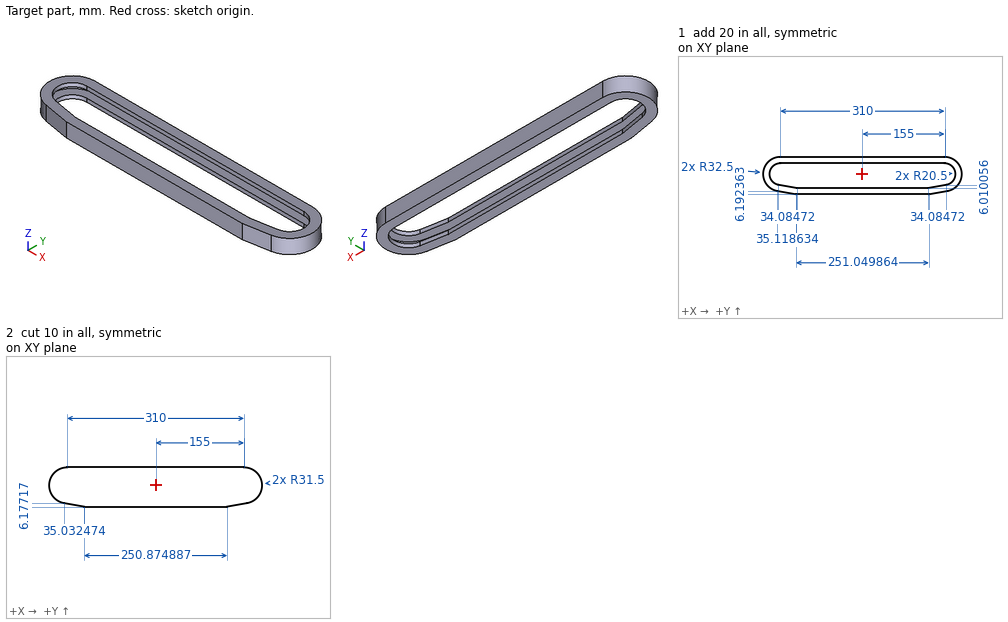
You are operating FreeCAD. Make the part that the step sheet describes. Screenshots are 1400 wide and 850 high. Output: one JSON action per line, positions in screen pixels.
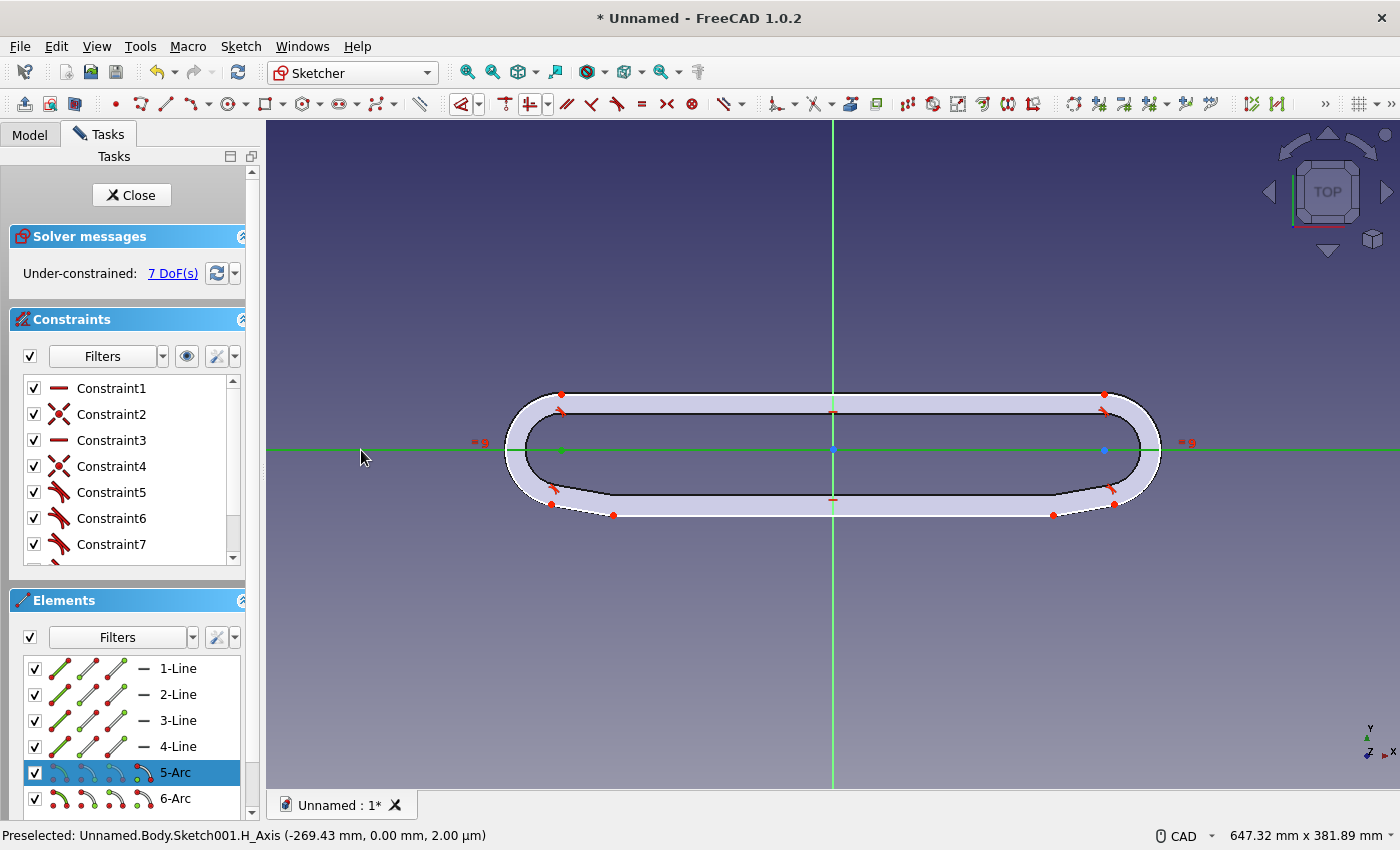
{"action": "left_click", "coordinate": [505, 104]}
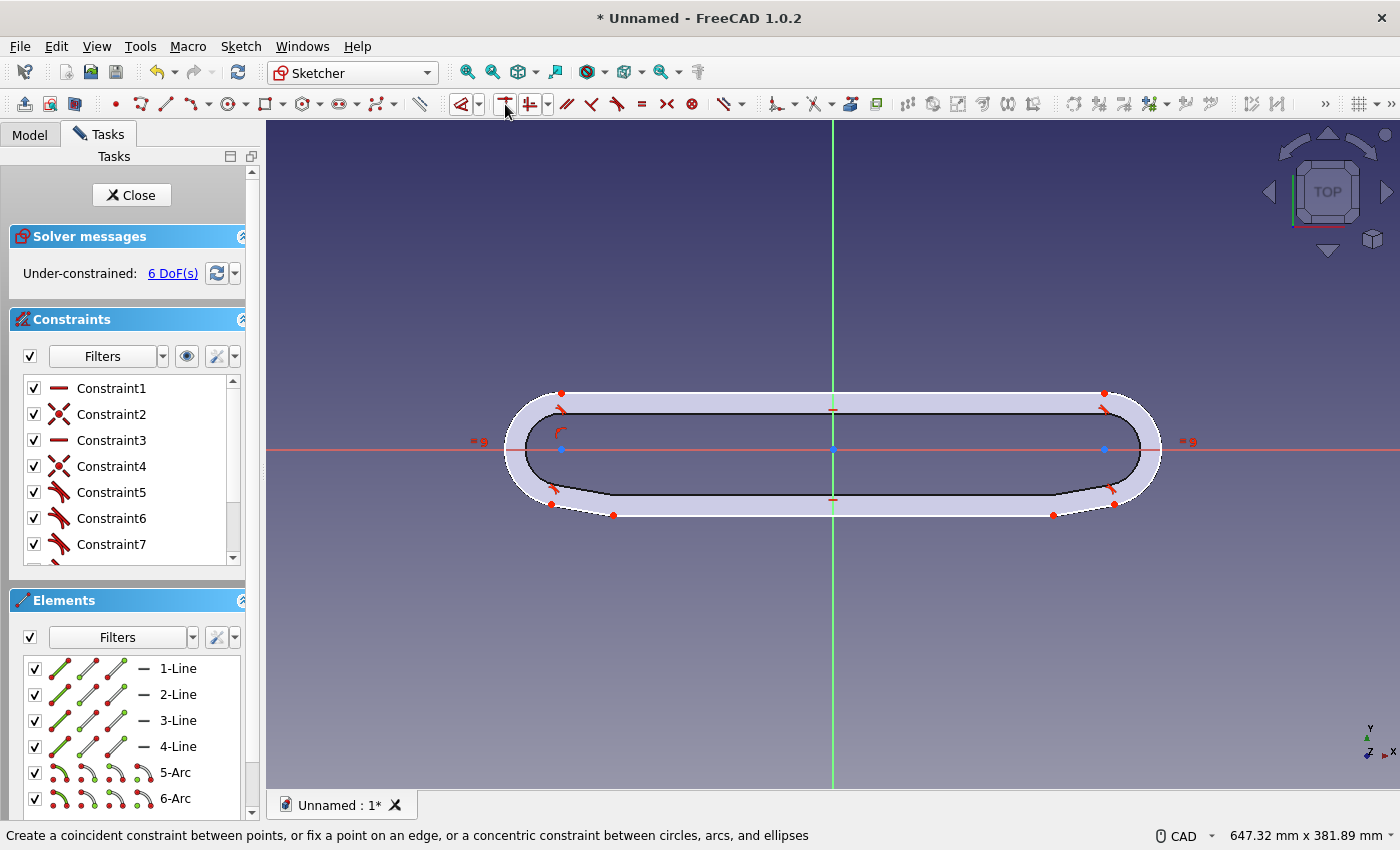
{"action": "left_click", "coordinate": [518, 414]}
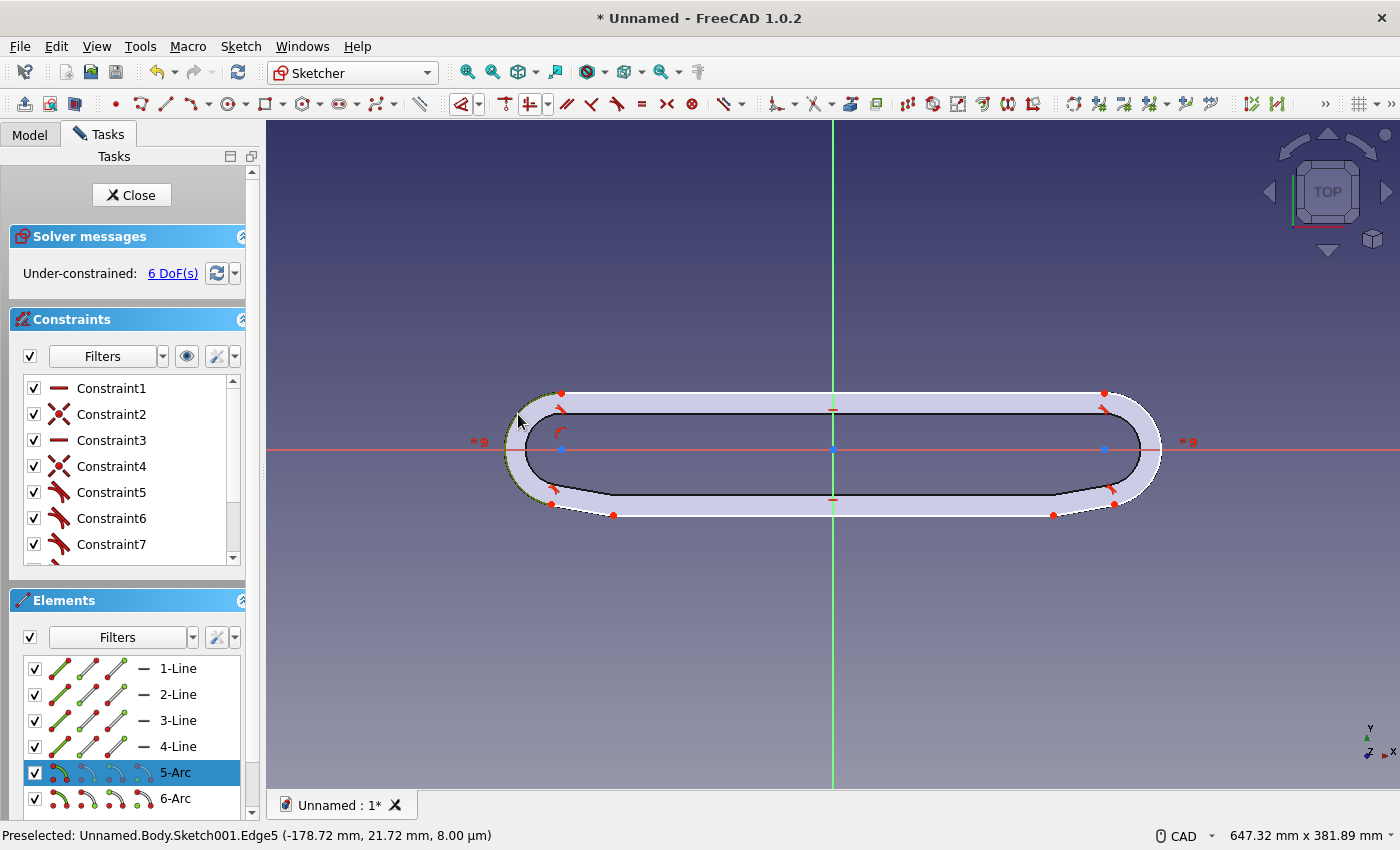
{"action": "key", "text": "k r"}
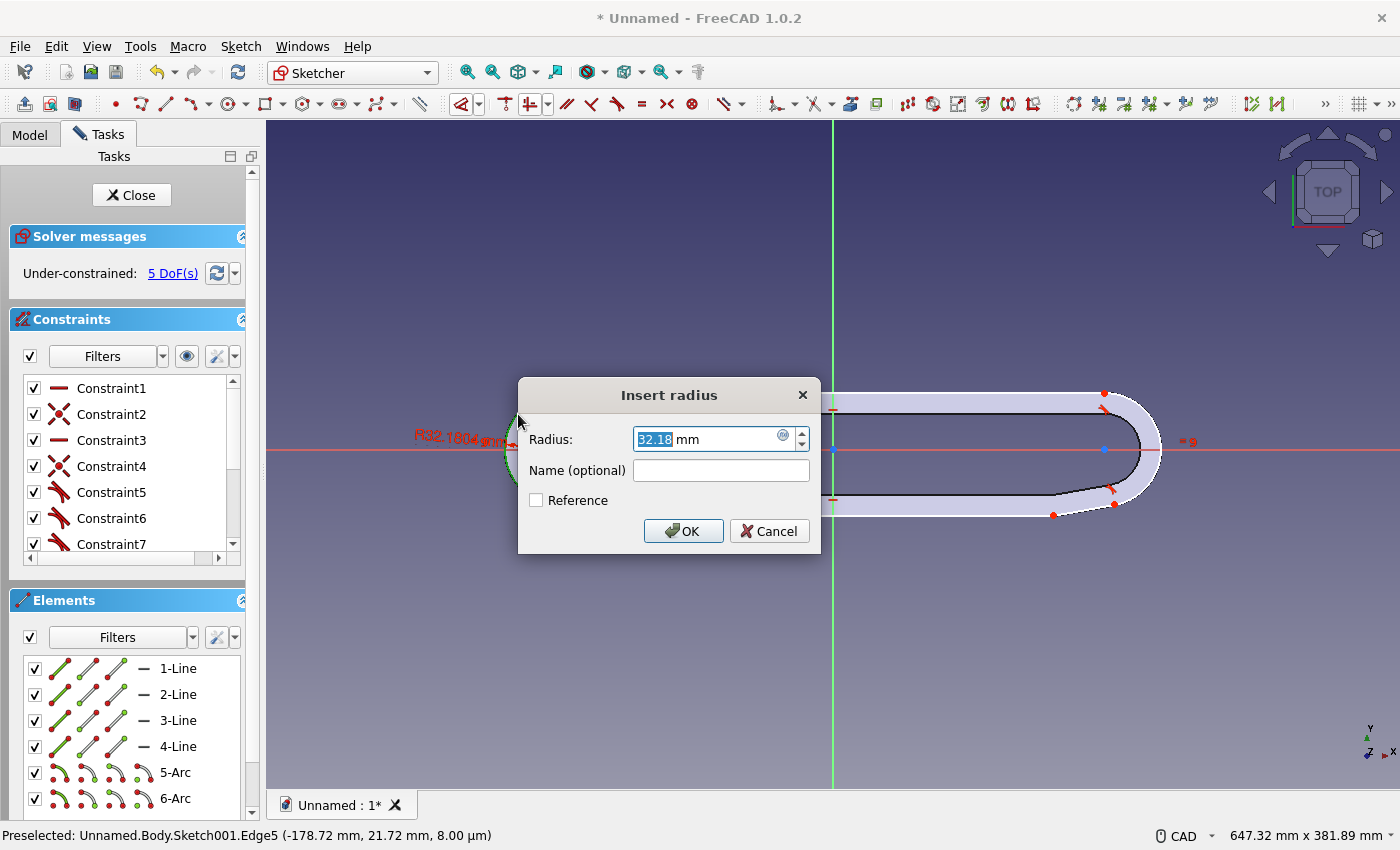
{"action": "type", "text": "31.5"}
{"action": "key", "text": "Return"}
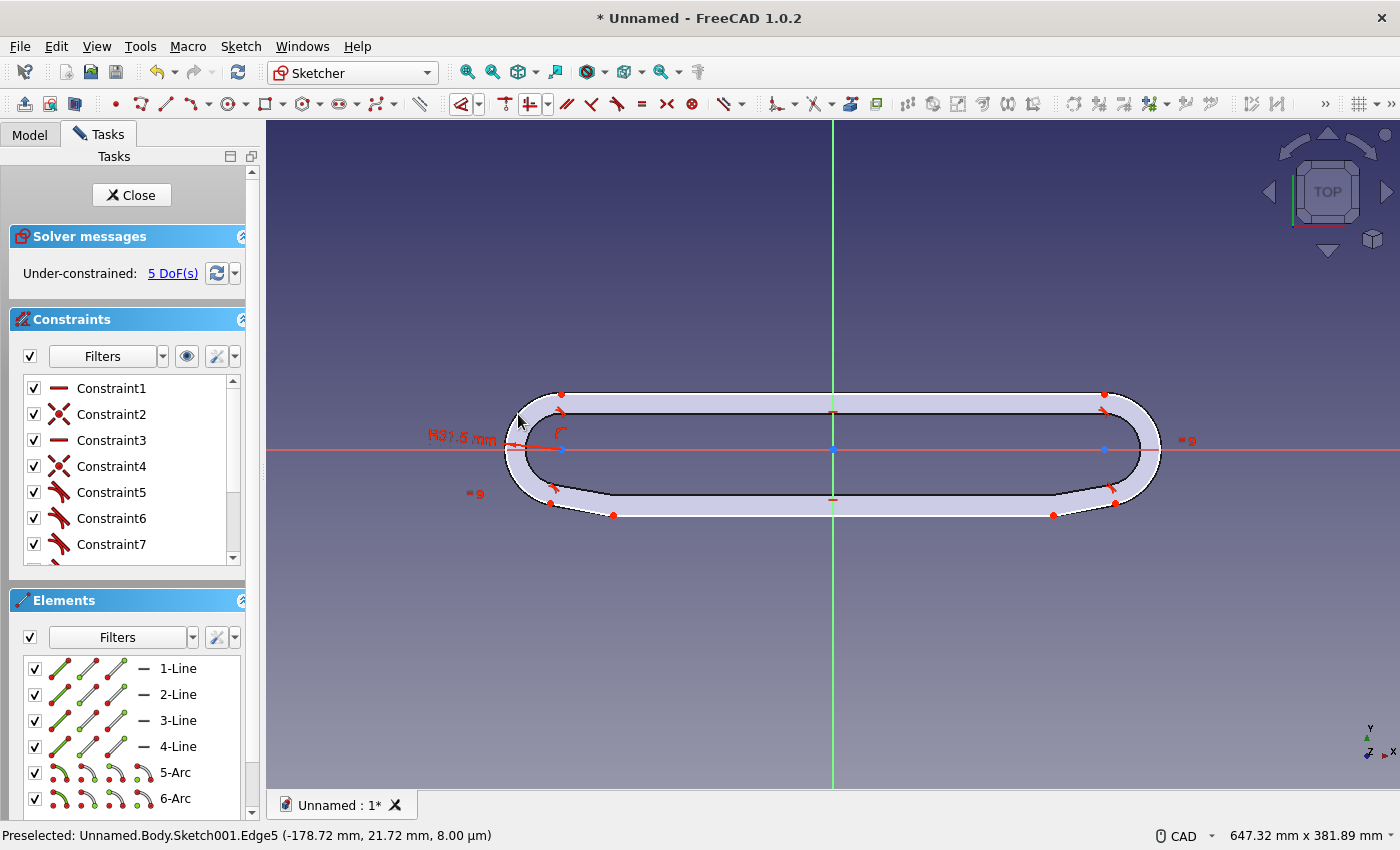
{"action": "left_click", "coordinate": [942, 394]}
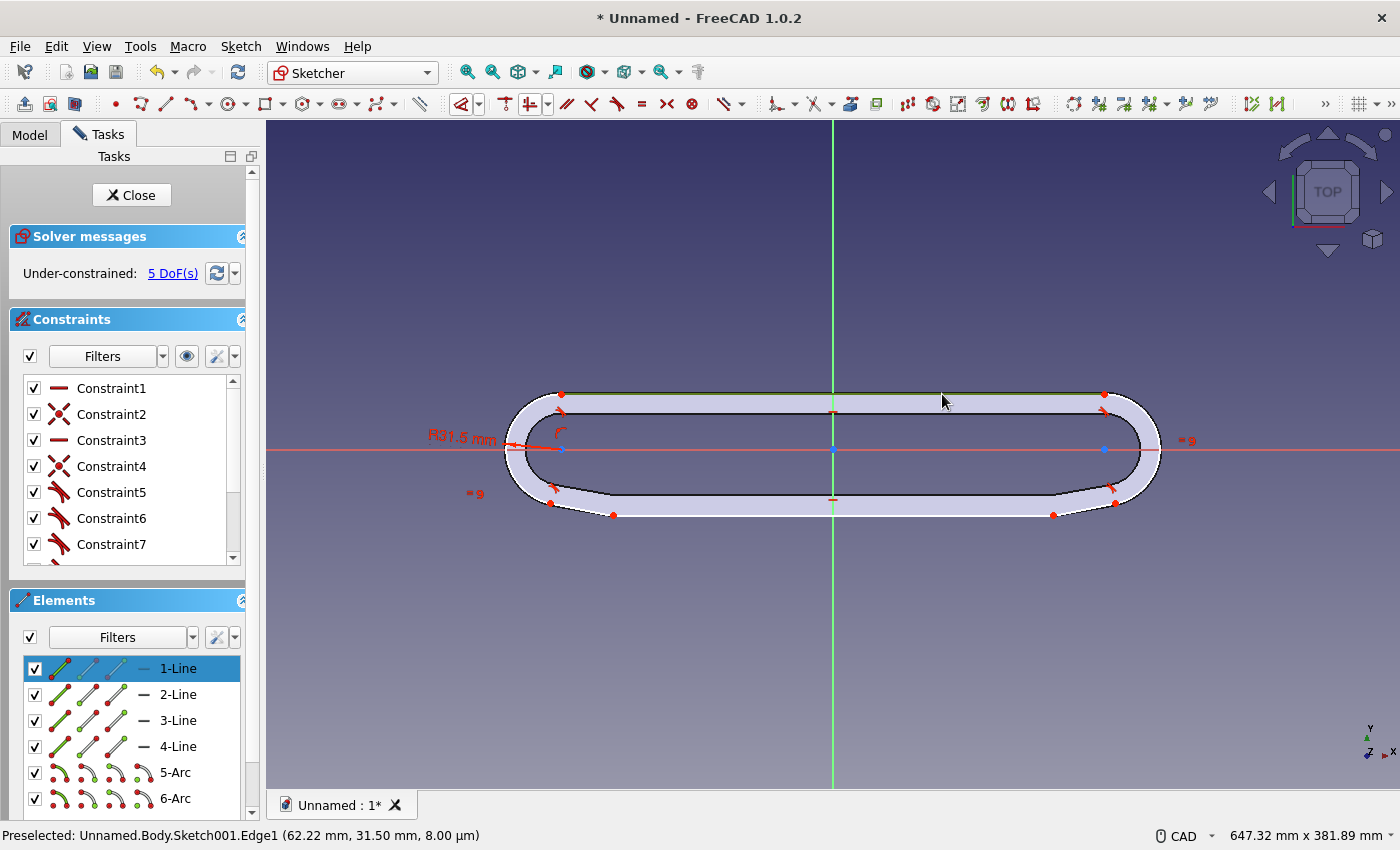
{"action": "key", "text": "l"}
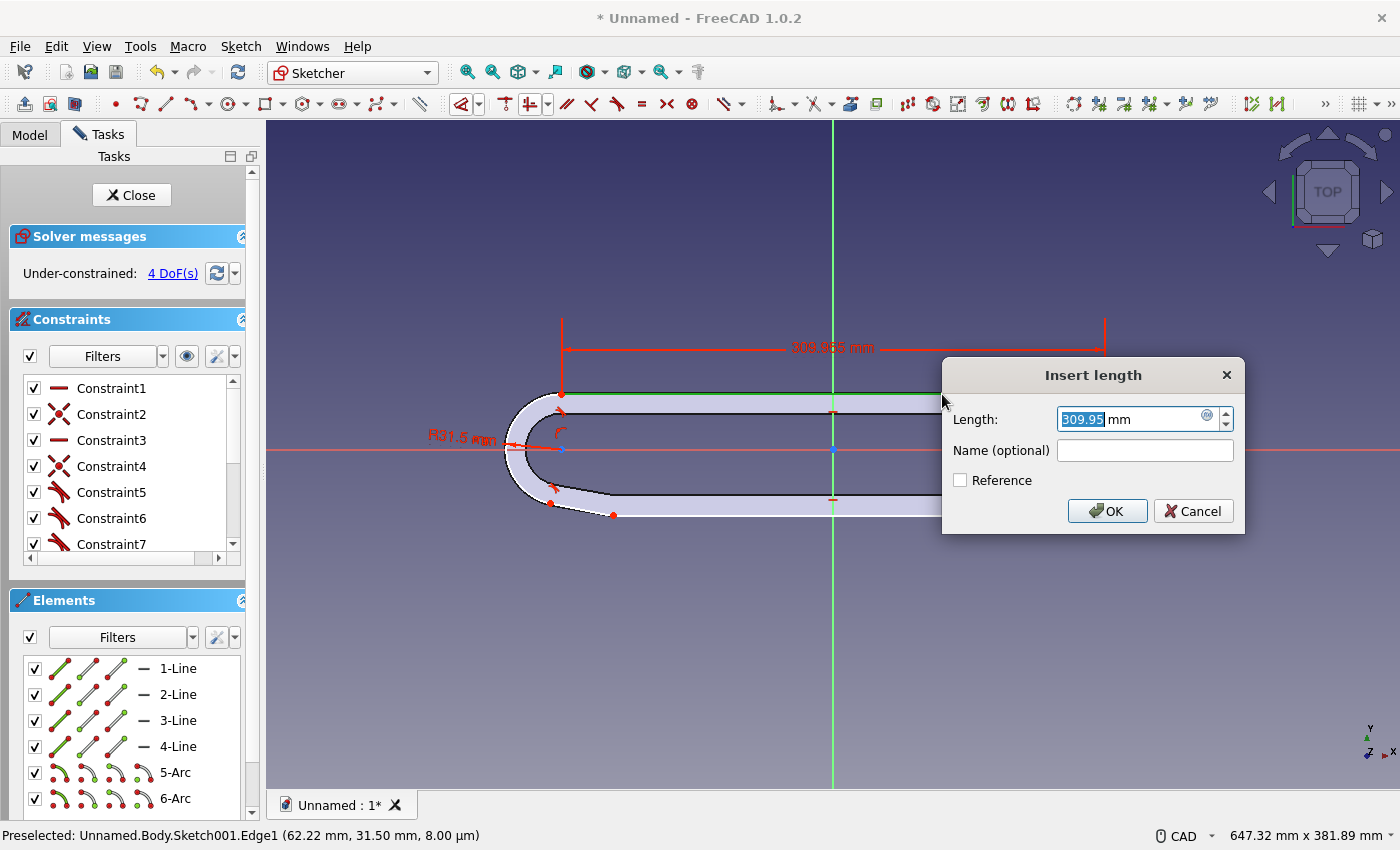
{"action": "type", "text": "310"}
{"action": "key", "text": "Return"}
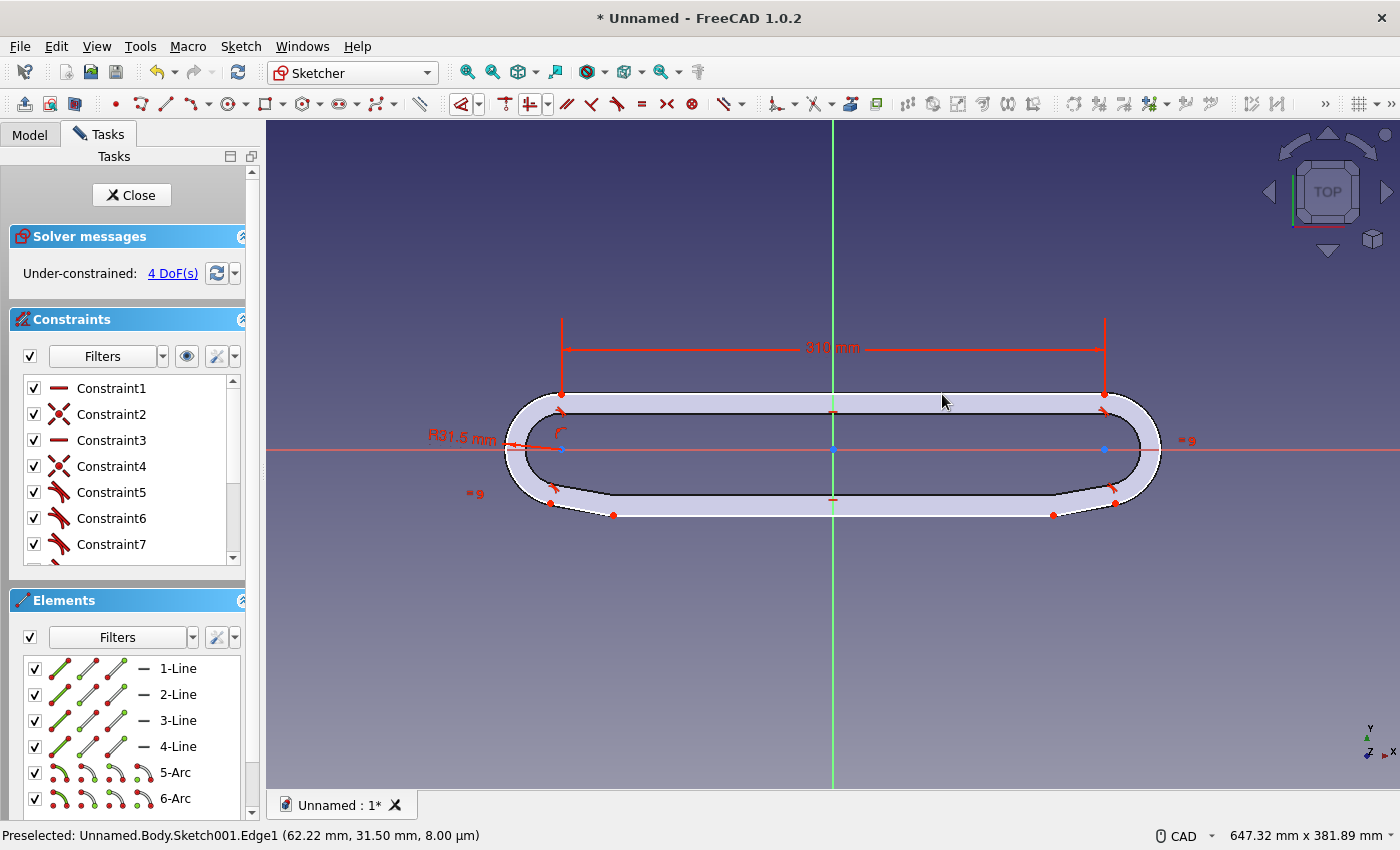
{"action": "left_click", "coordinate": [1105, 394]}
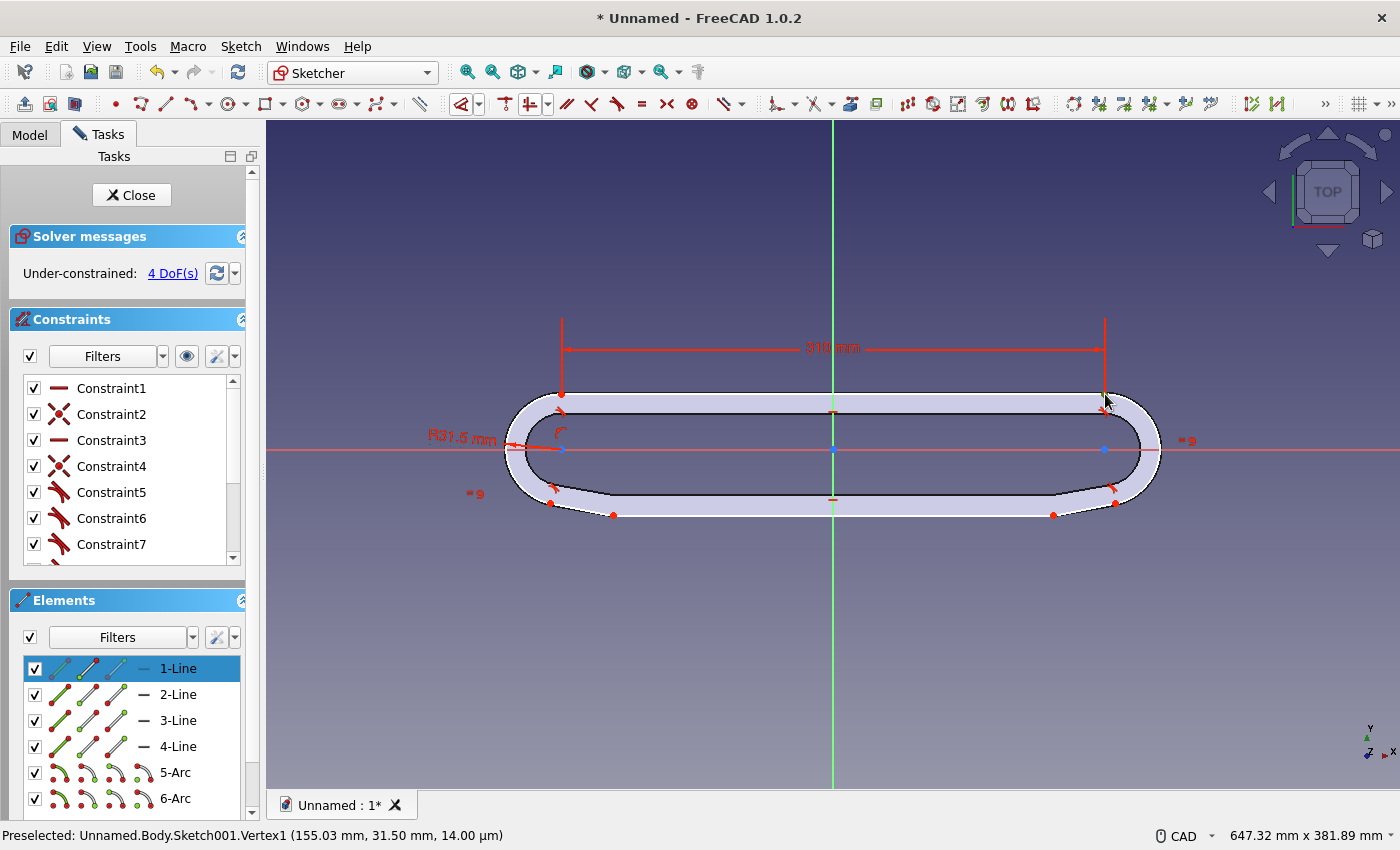
{"action": "key", "text": "l"}